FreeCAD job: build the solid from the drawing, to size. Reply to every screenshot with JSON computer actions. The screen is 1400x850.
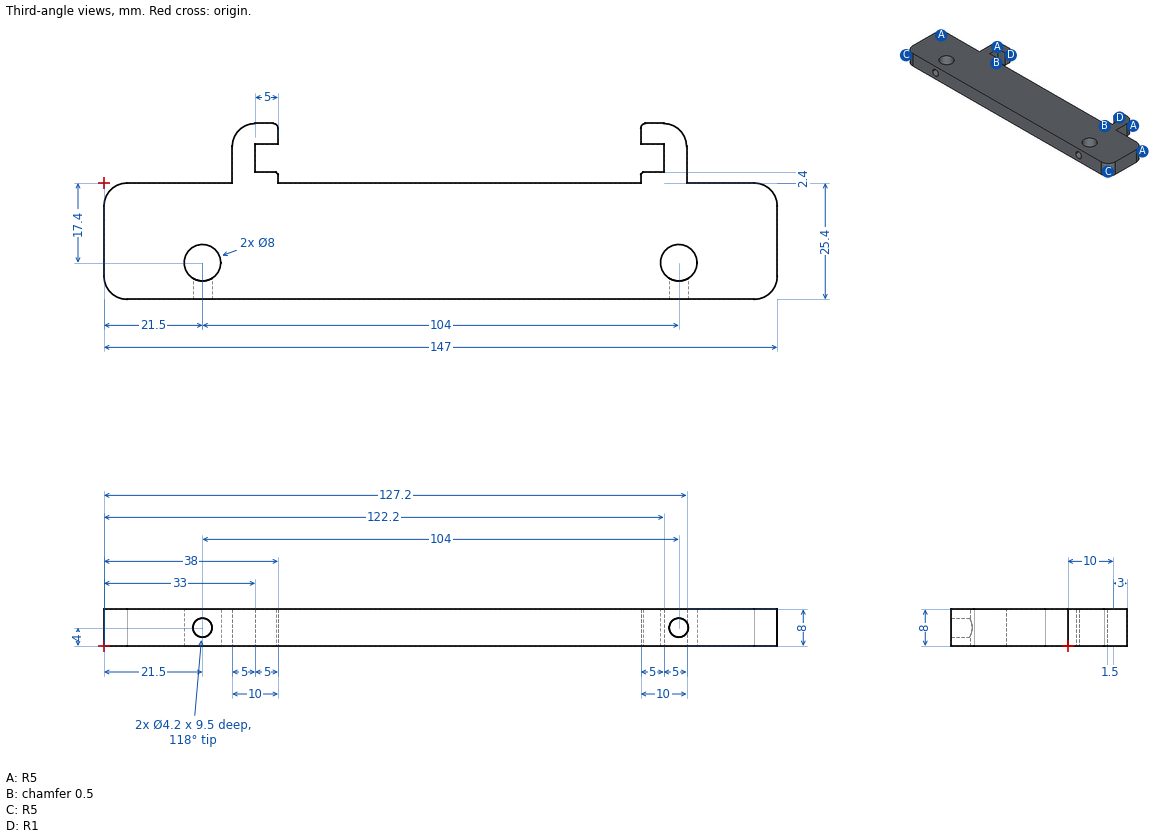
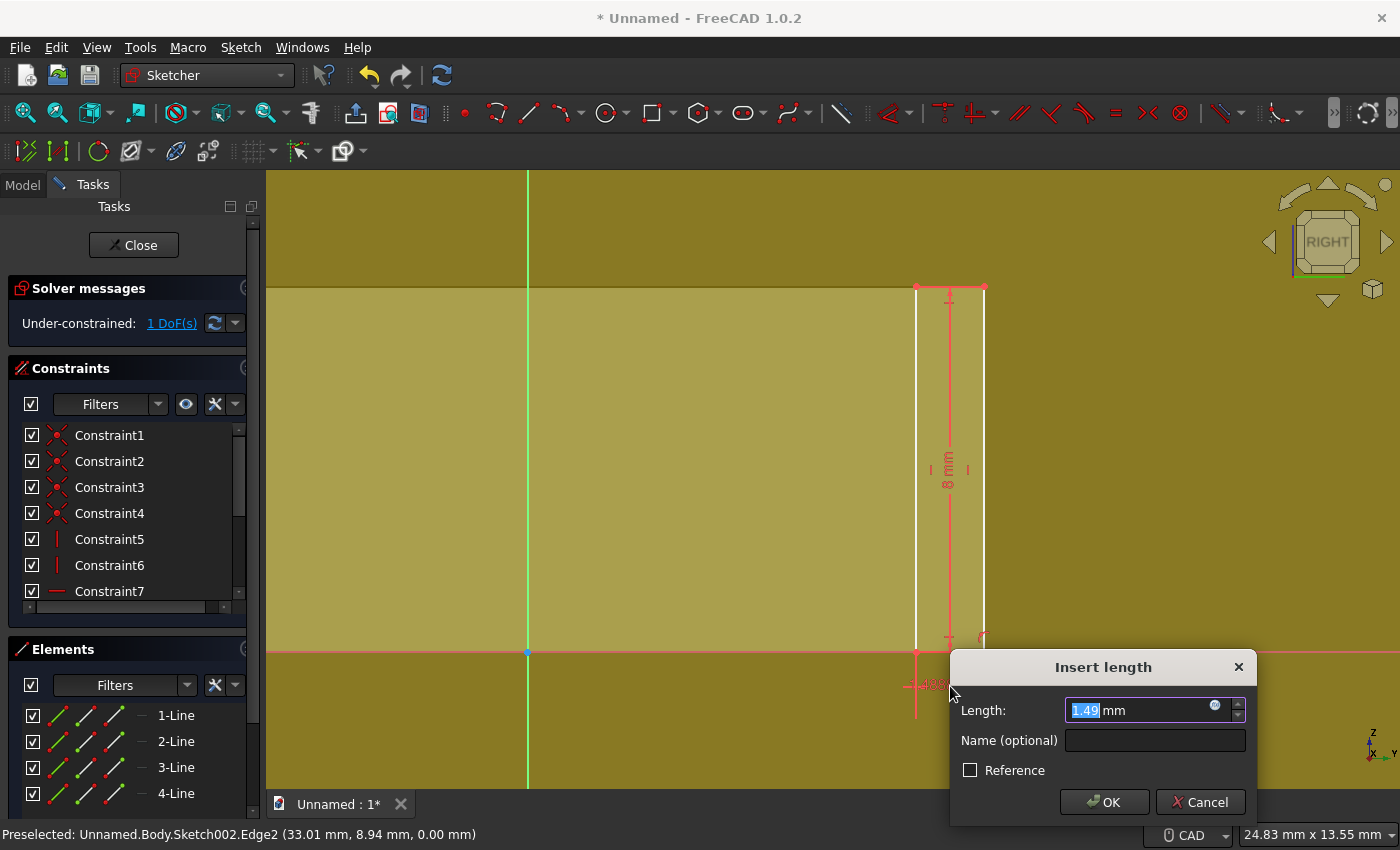
{"action": "type", "text": "1.5"}
{"action": "key", "text": "Return"}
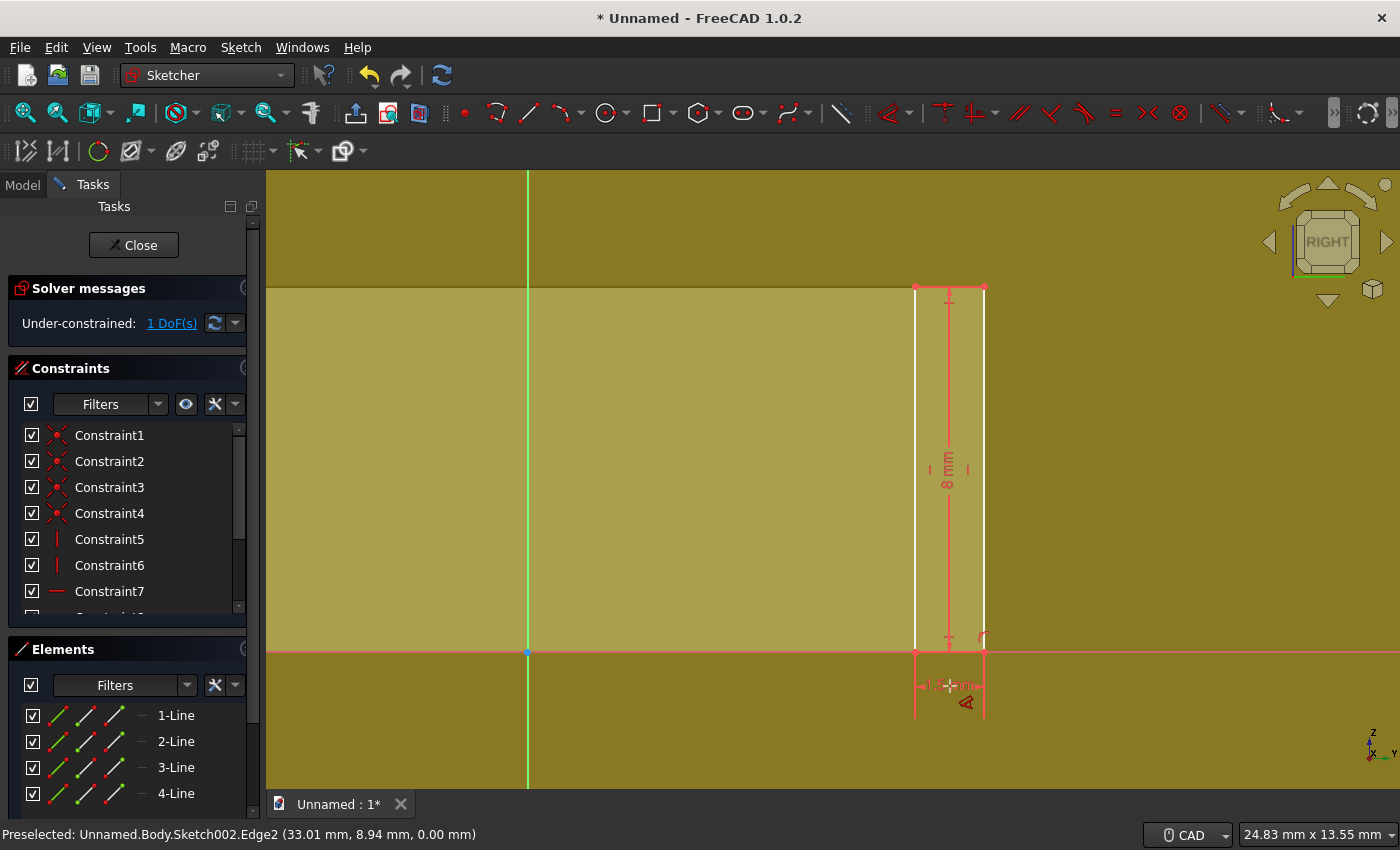
{"action": "left_click", "coordinate": [984, 652]}
{"action": "left_click", "coordinate": [756, 686]}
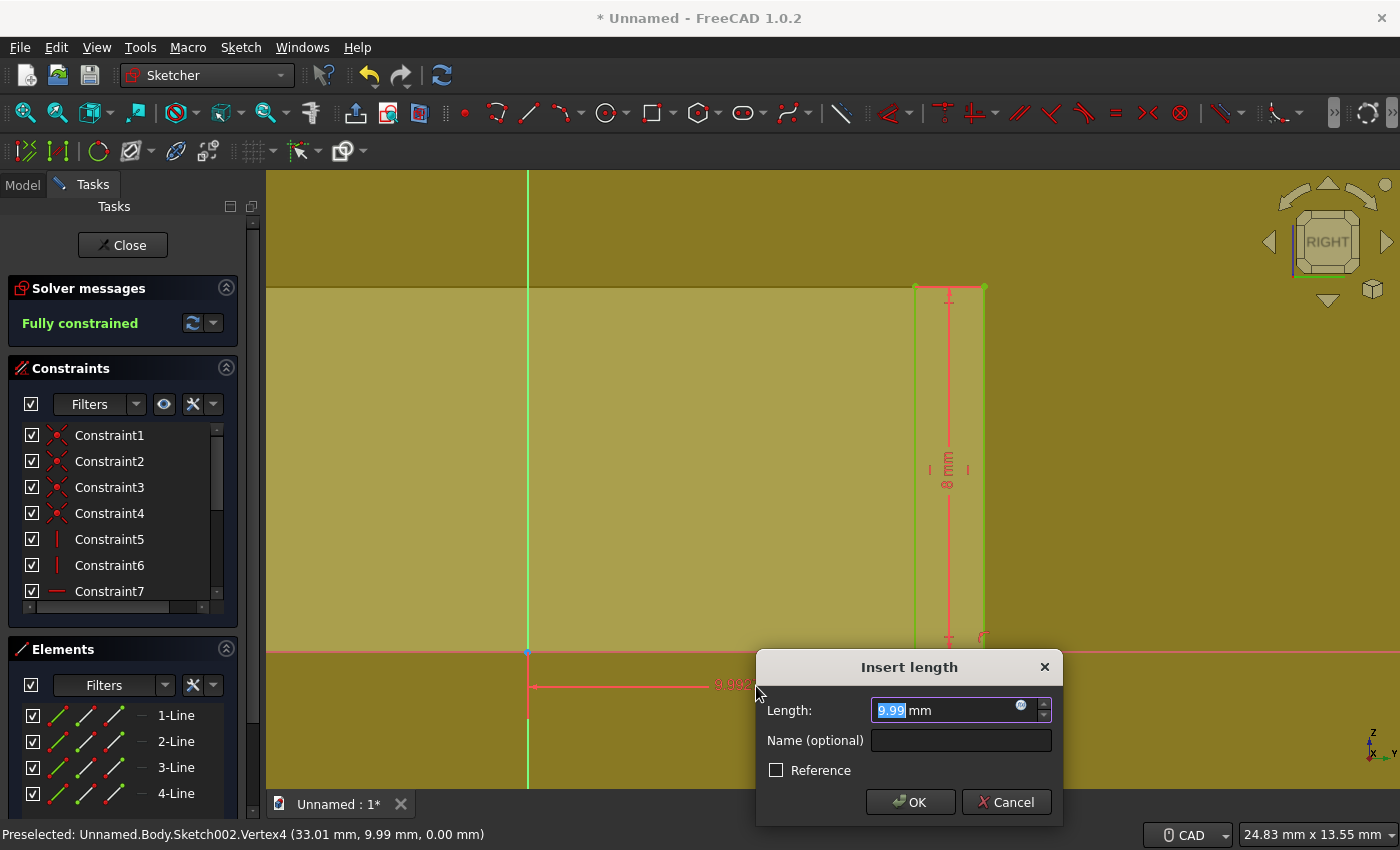
{"action": "type", "text": "10"}
{"action": "key", "text": "Return"}
{"action": "key", "text": "Escape"}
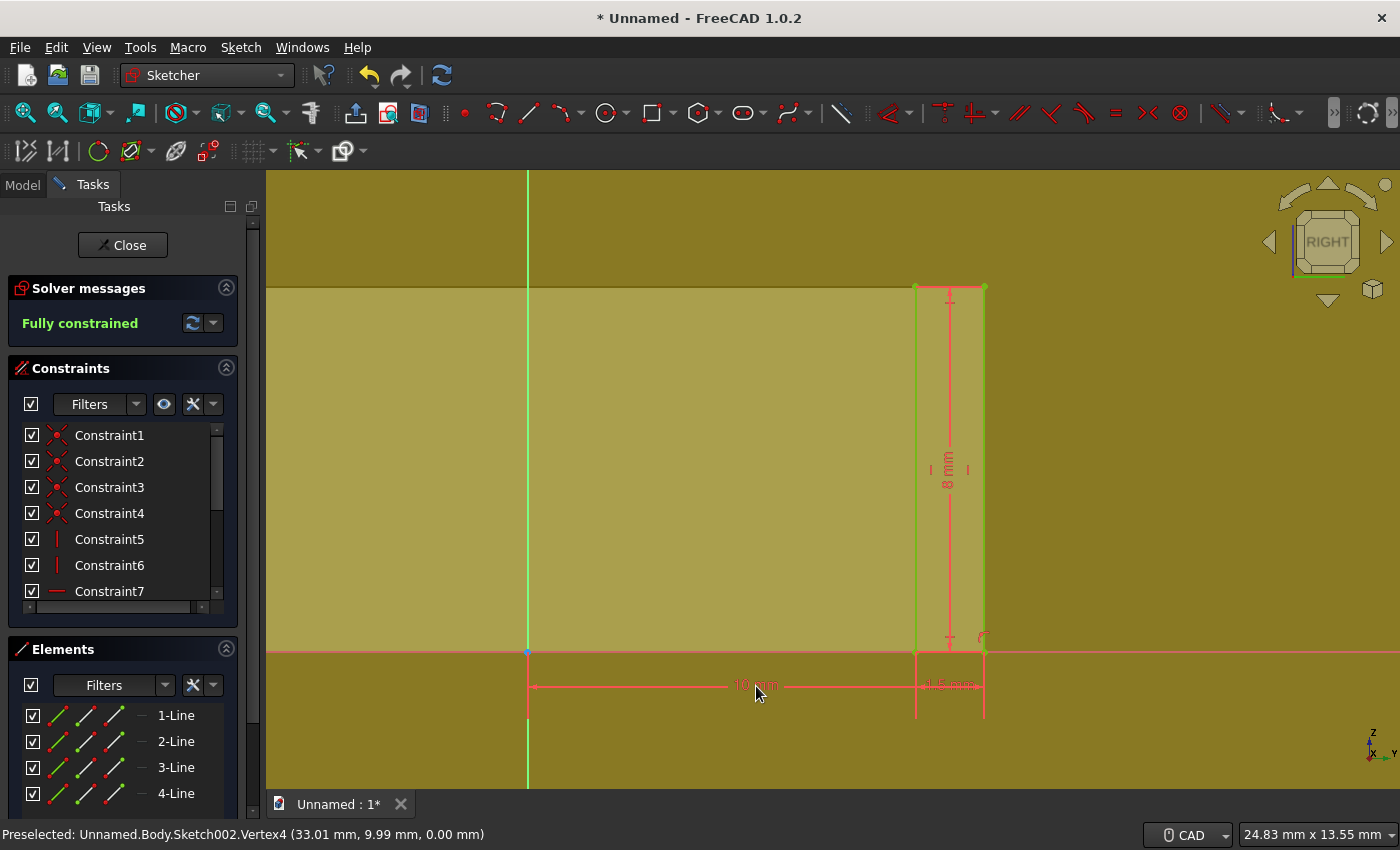
{"action": "left_click", "coordinate": [123, 245]}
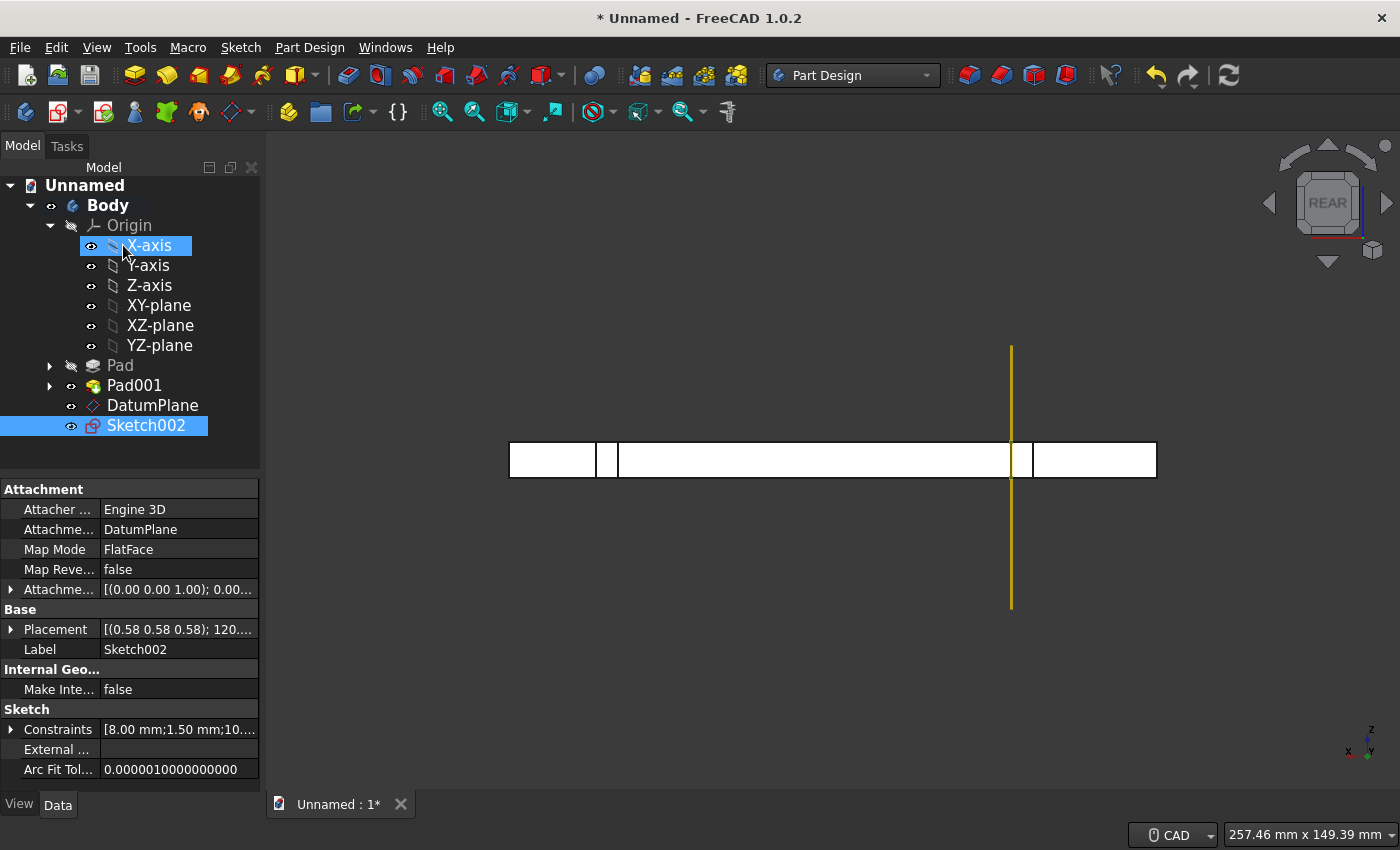
{"action": "left_click", "coordinate": [136, 76]}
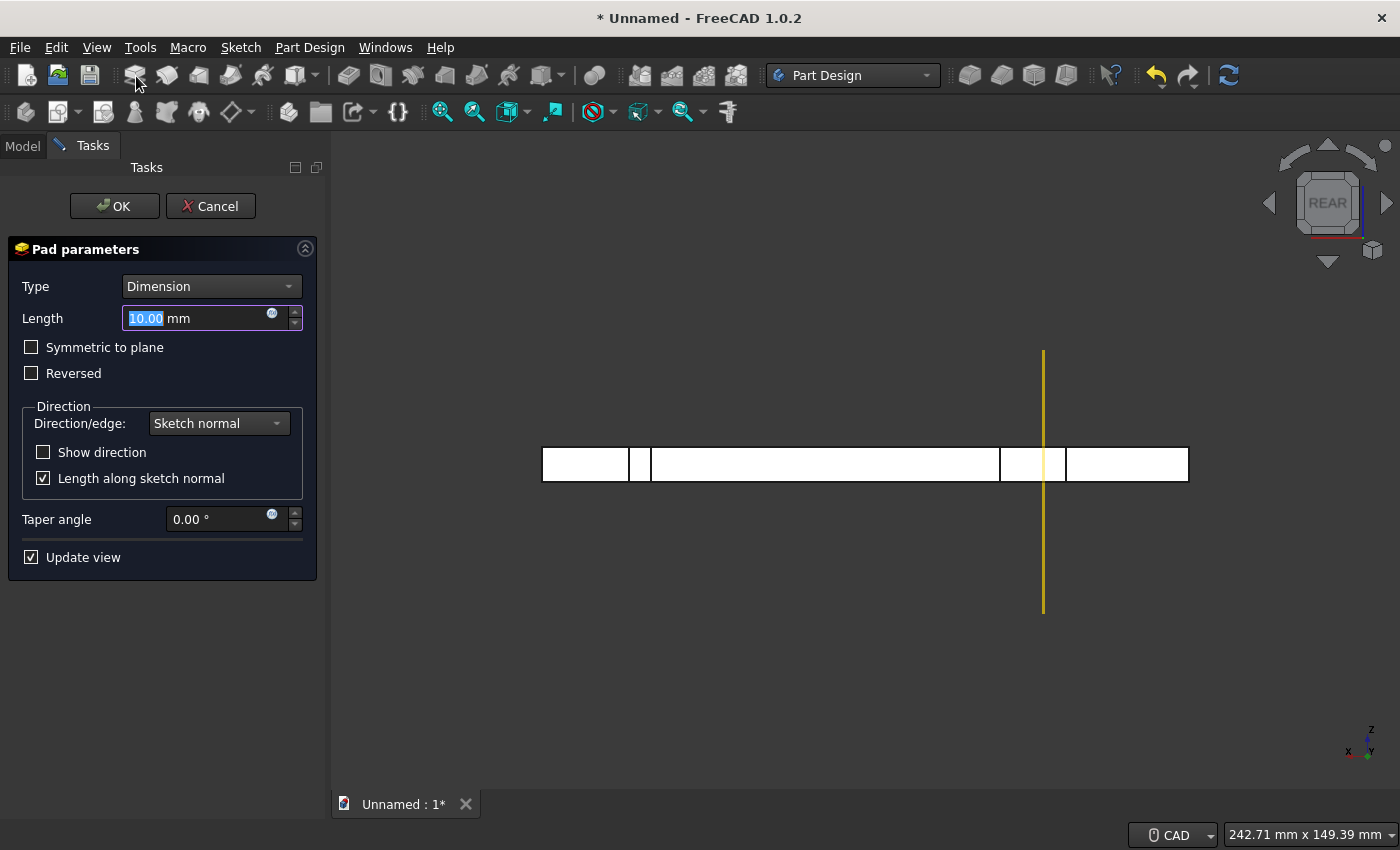
{"action": "type", "text": "5"}
{"action": "key", "text": "Tab"}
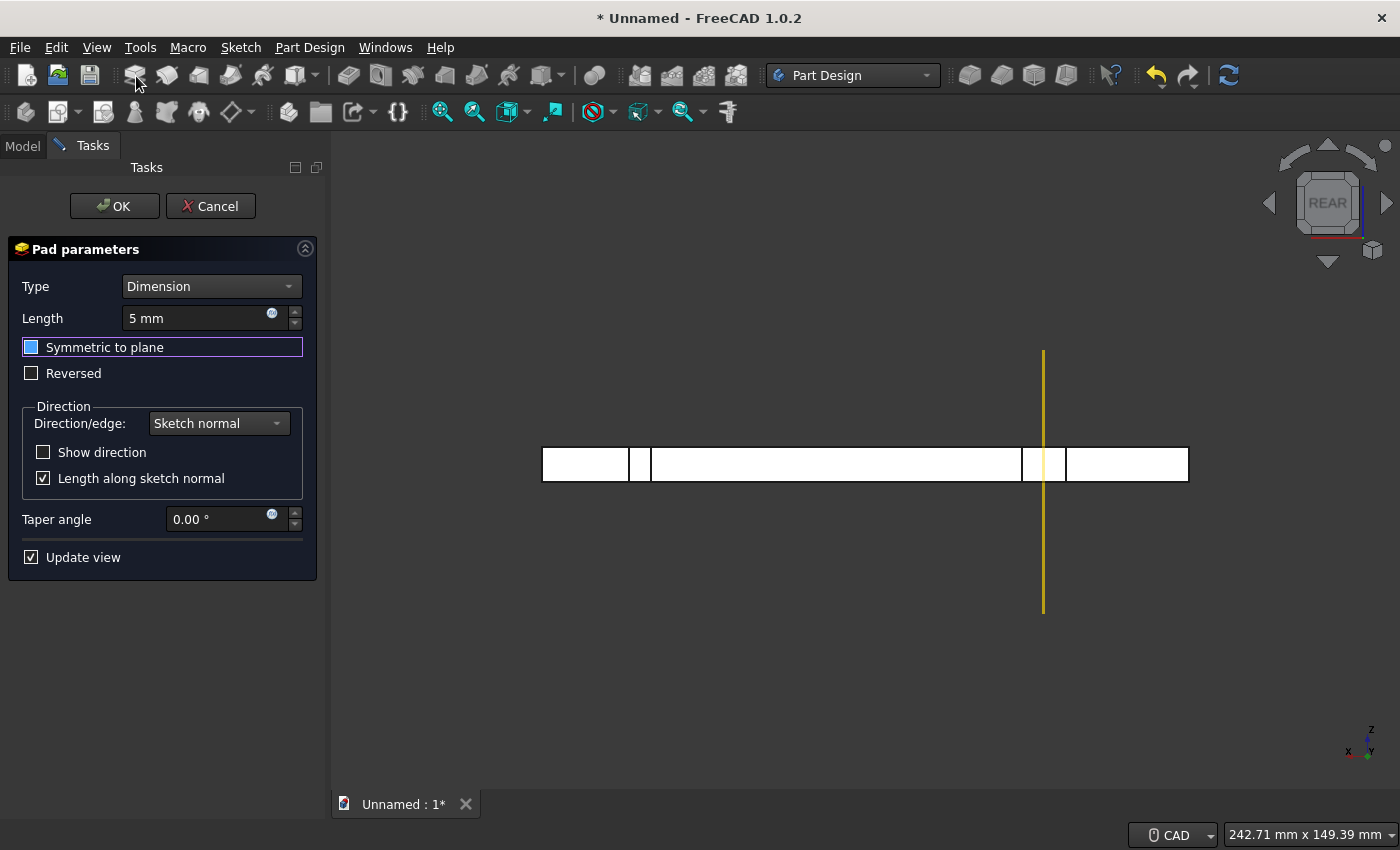
{"action": "left_click", "coordinate": [115, 206]}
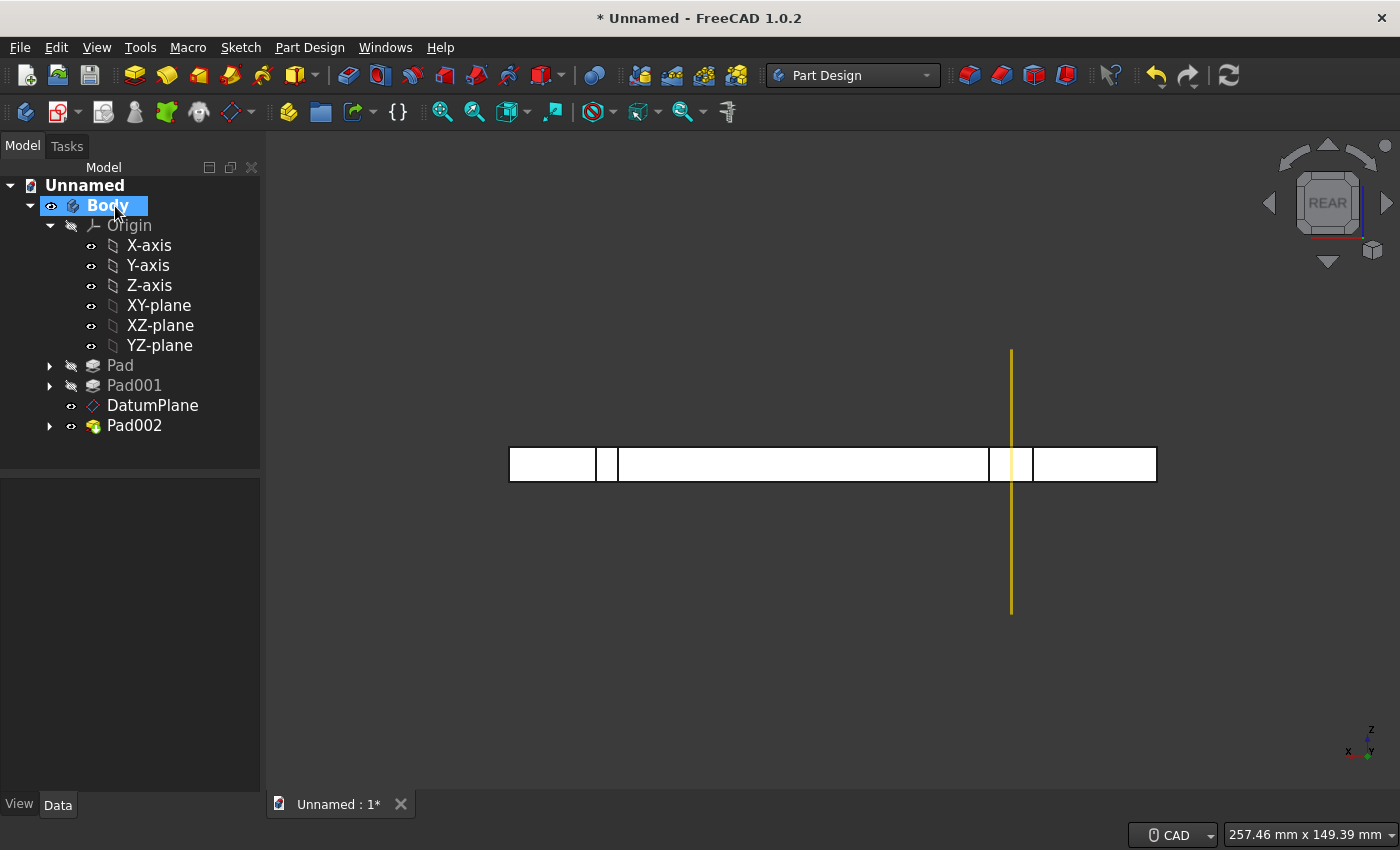
{"action": "left_click", "coordinate": [116, 406]}
{"action": "key", "text": "space"}